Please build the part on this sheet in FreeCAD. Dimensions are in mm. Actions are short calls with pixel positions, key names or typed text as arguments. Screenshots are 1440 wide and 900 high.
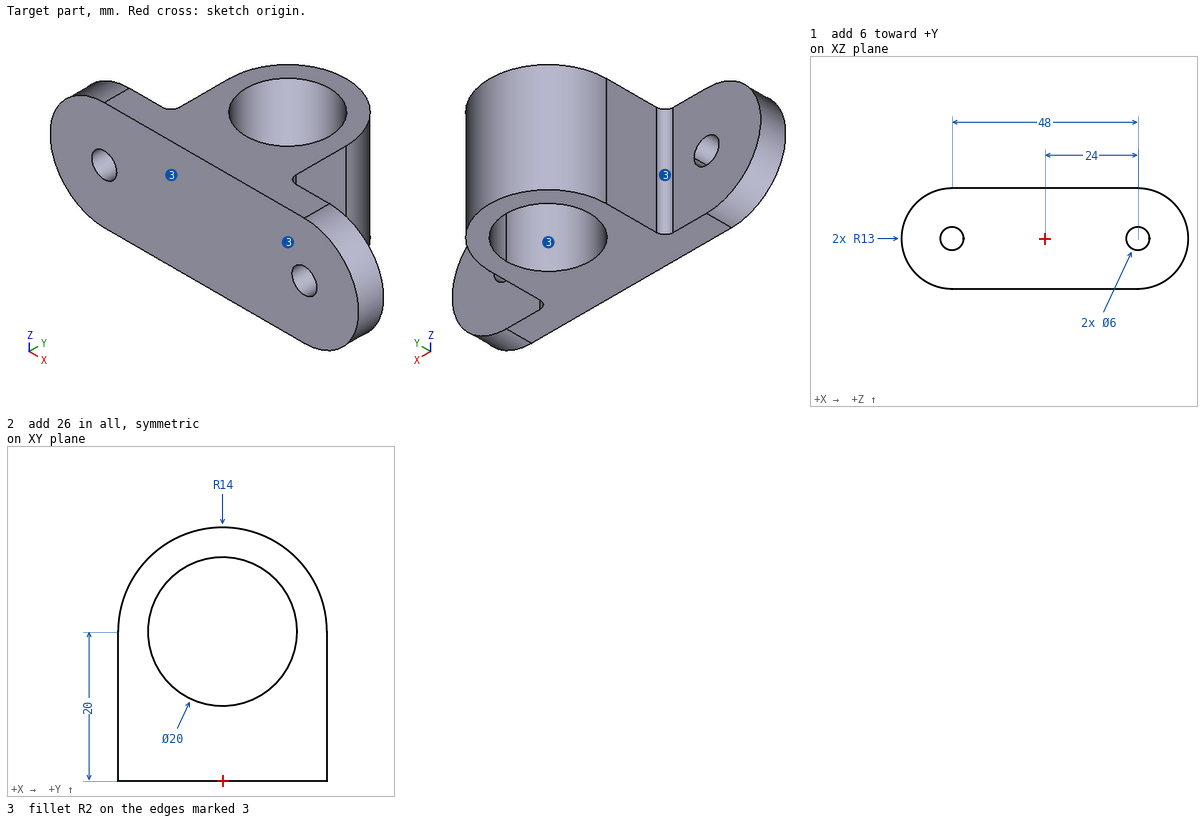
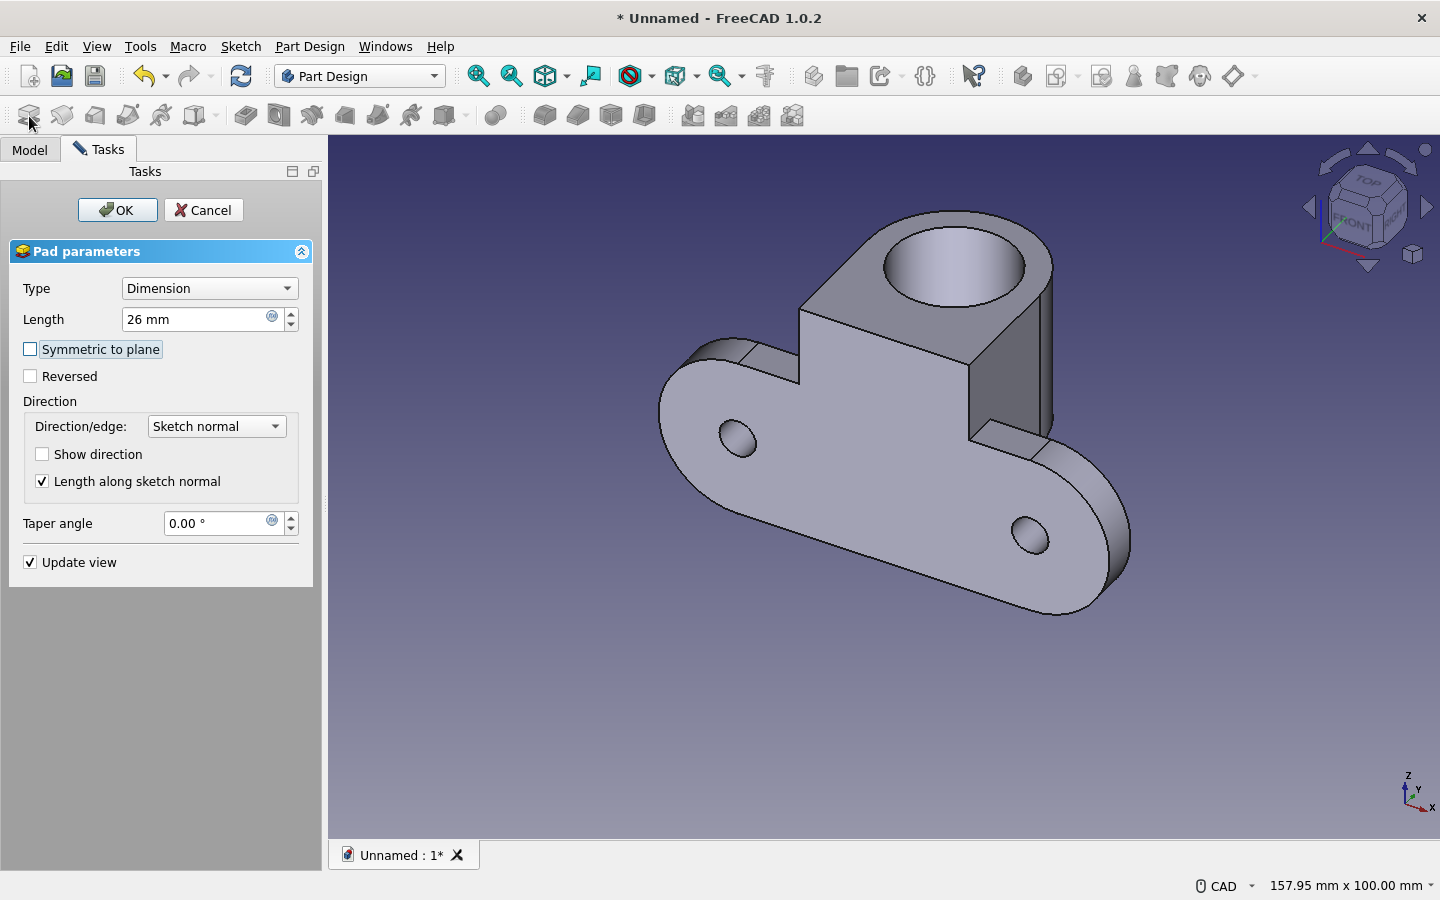
click(31, 349)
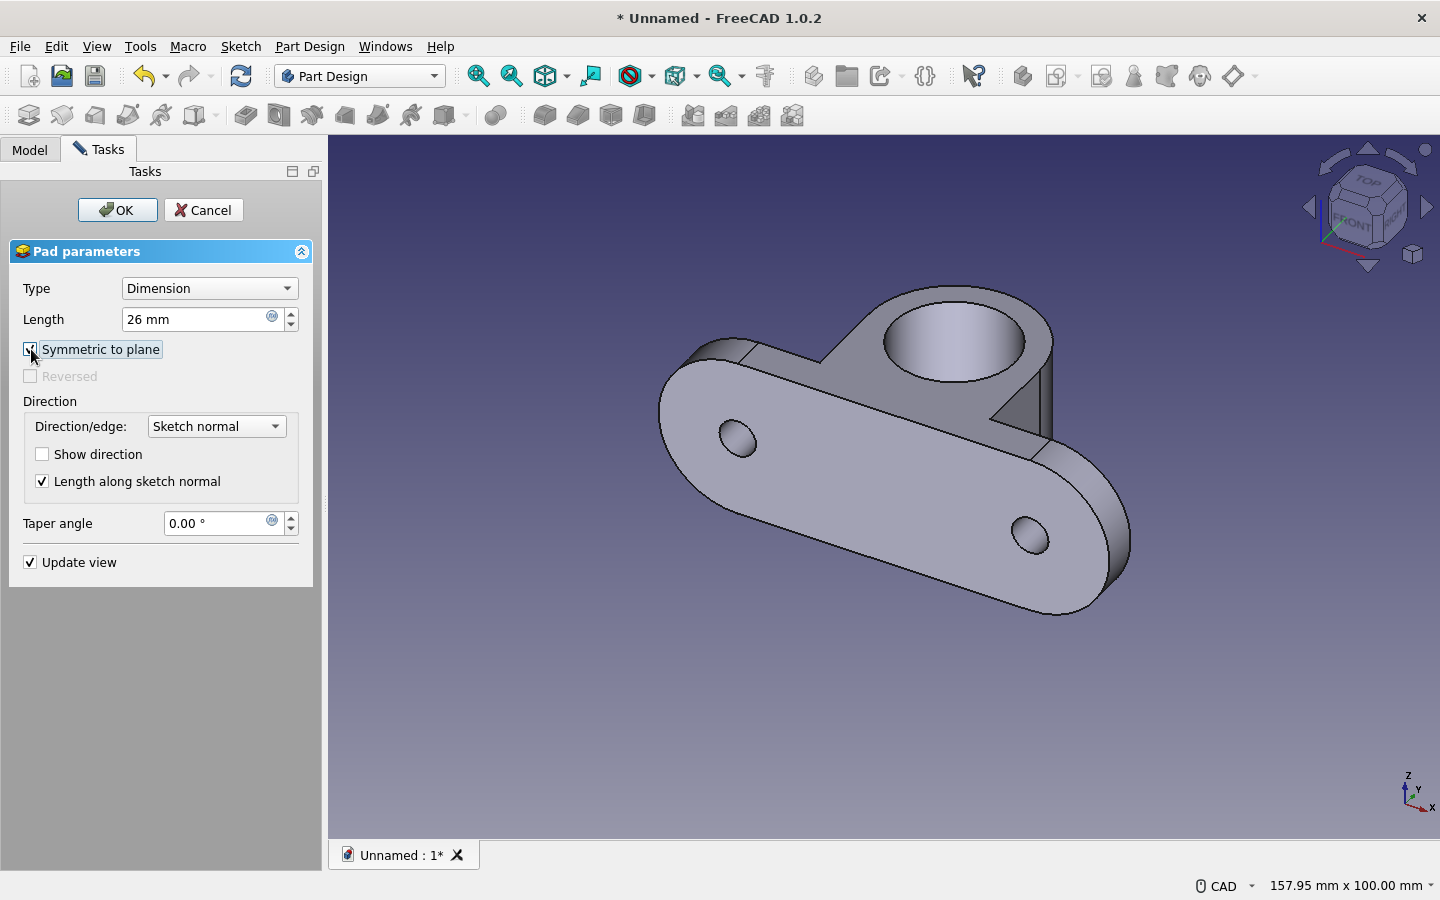
click(118, 210)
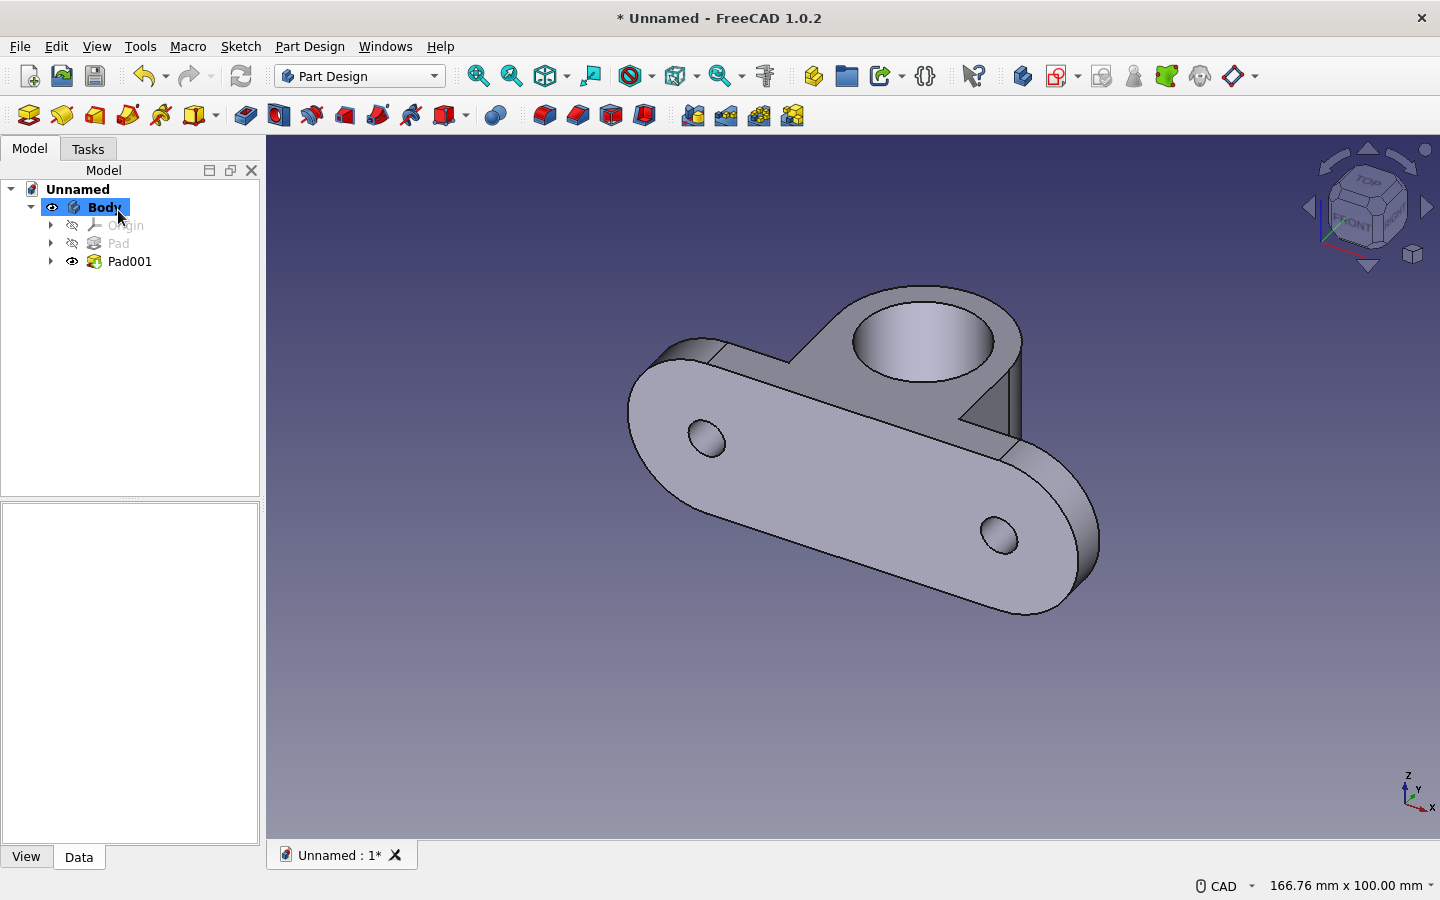
key(0)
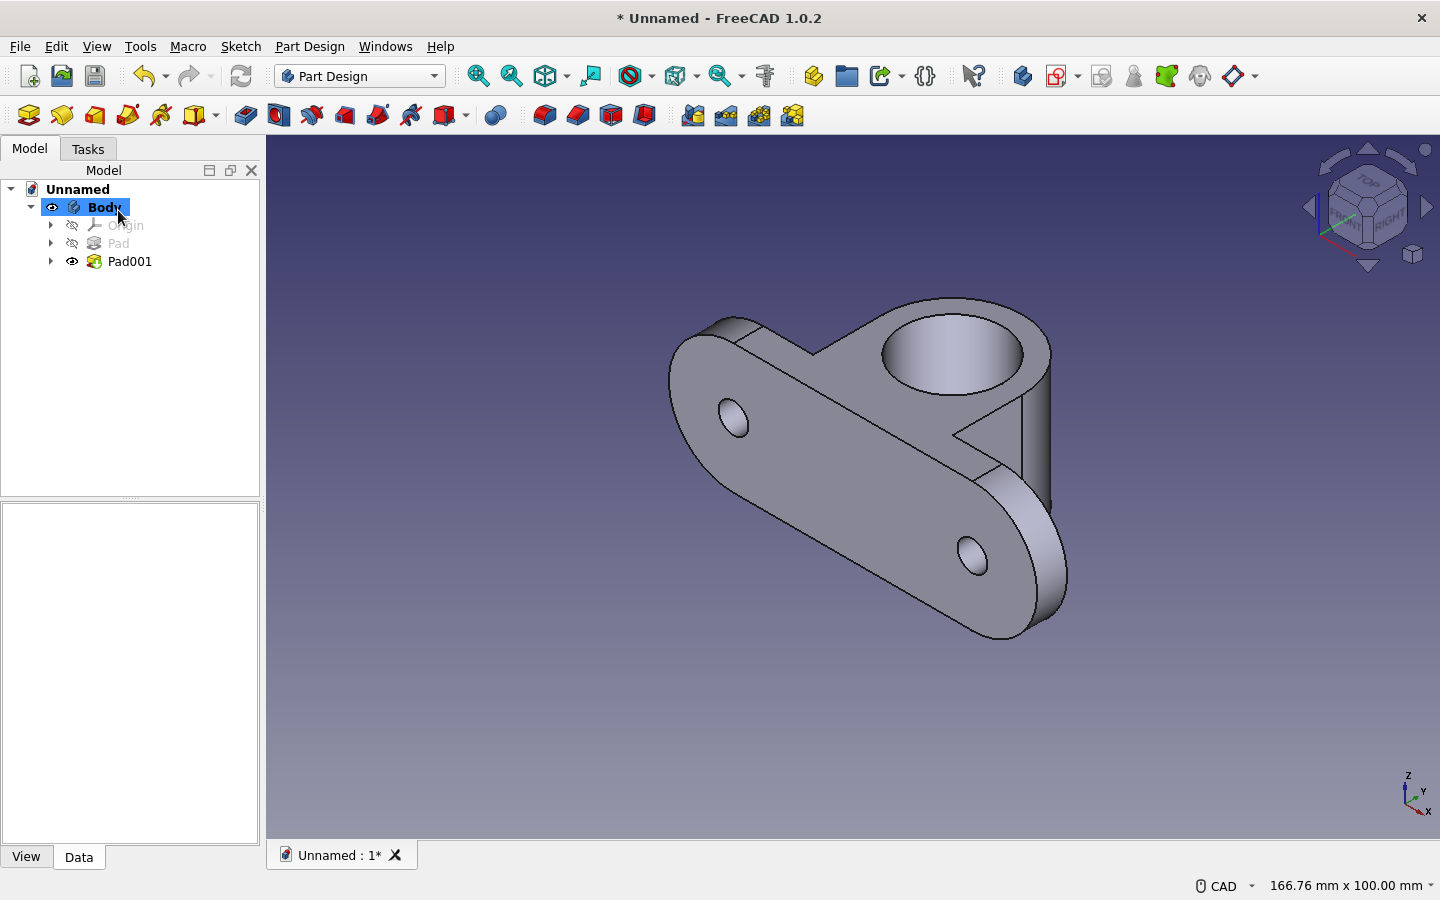
key(2)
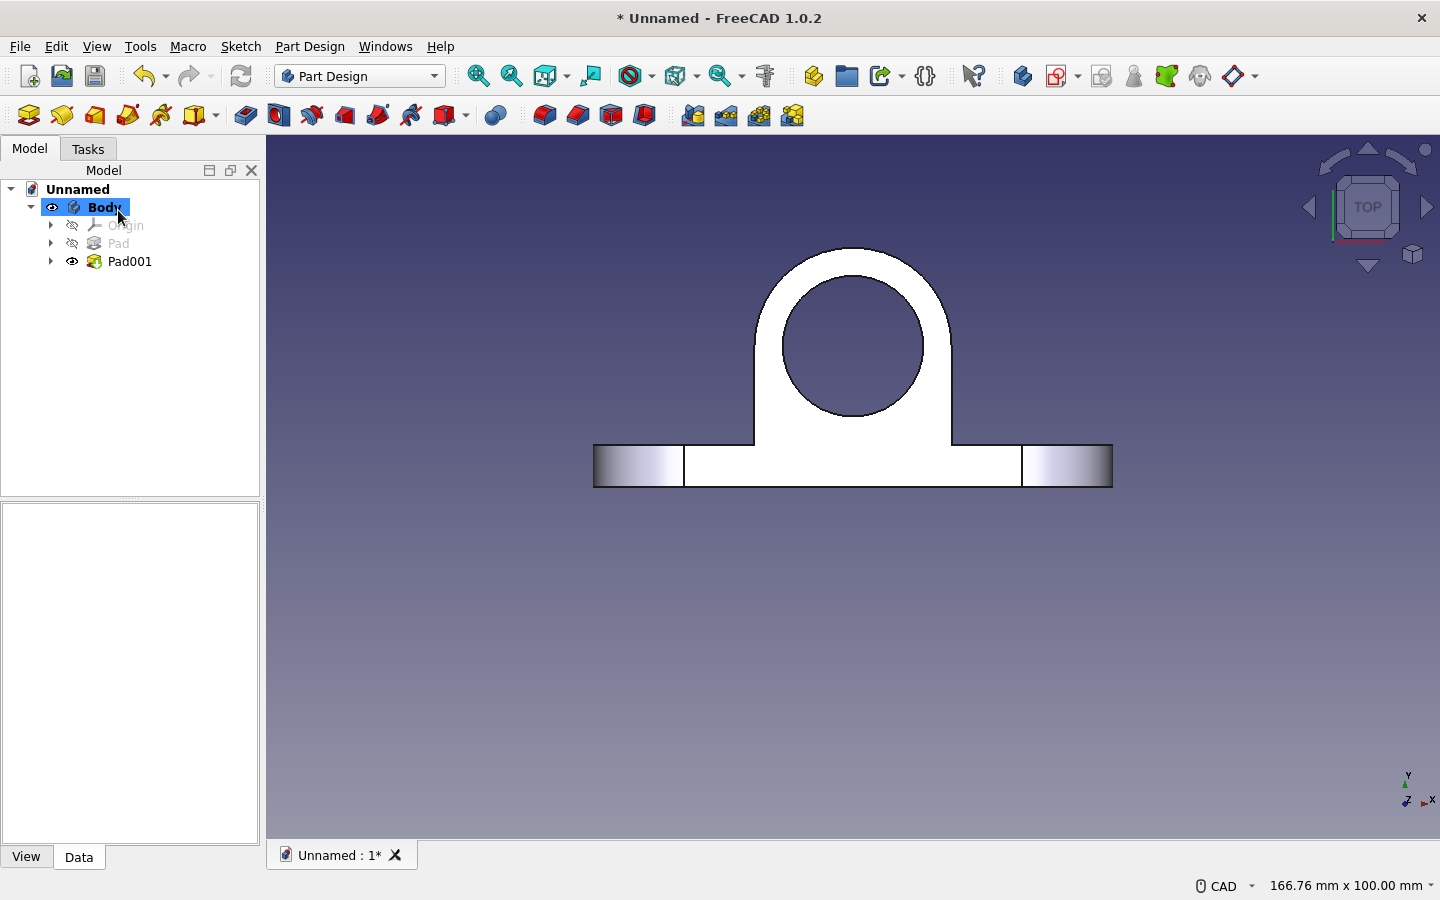
click(479, 76)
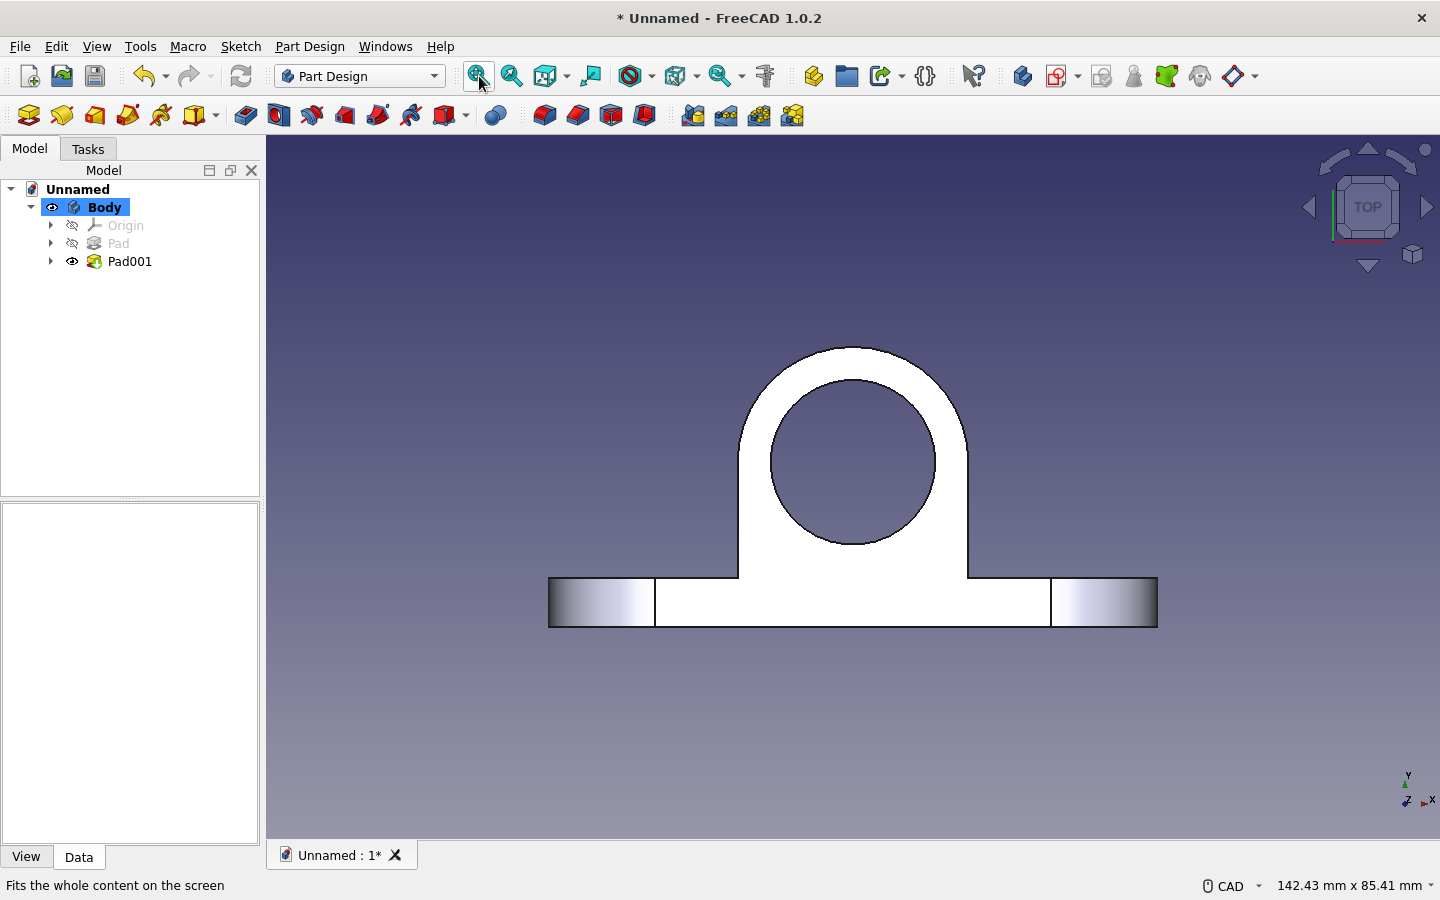
key(1)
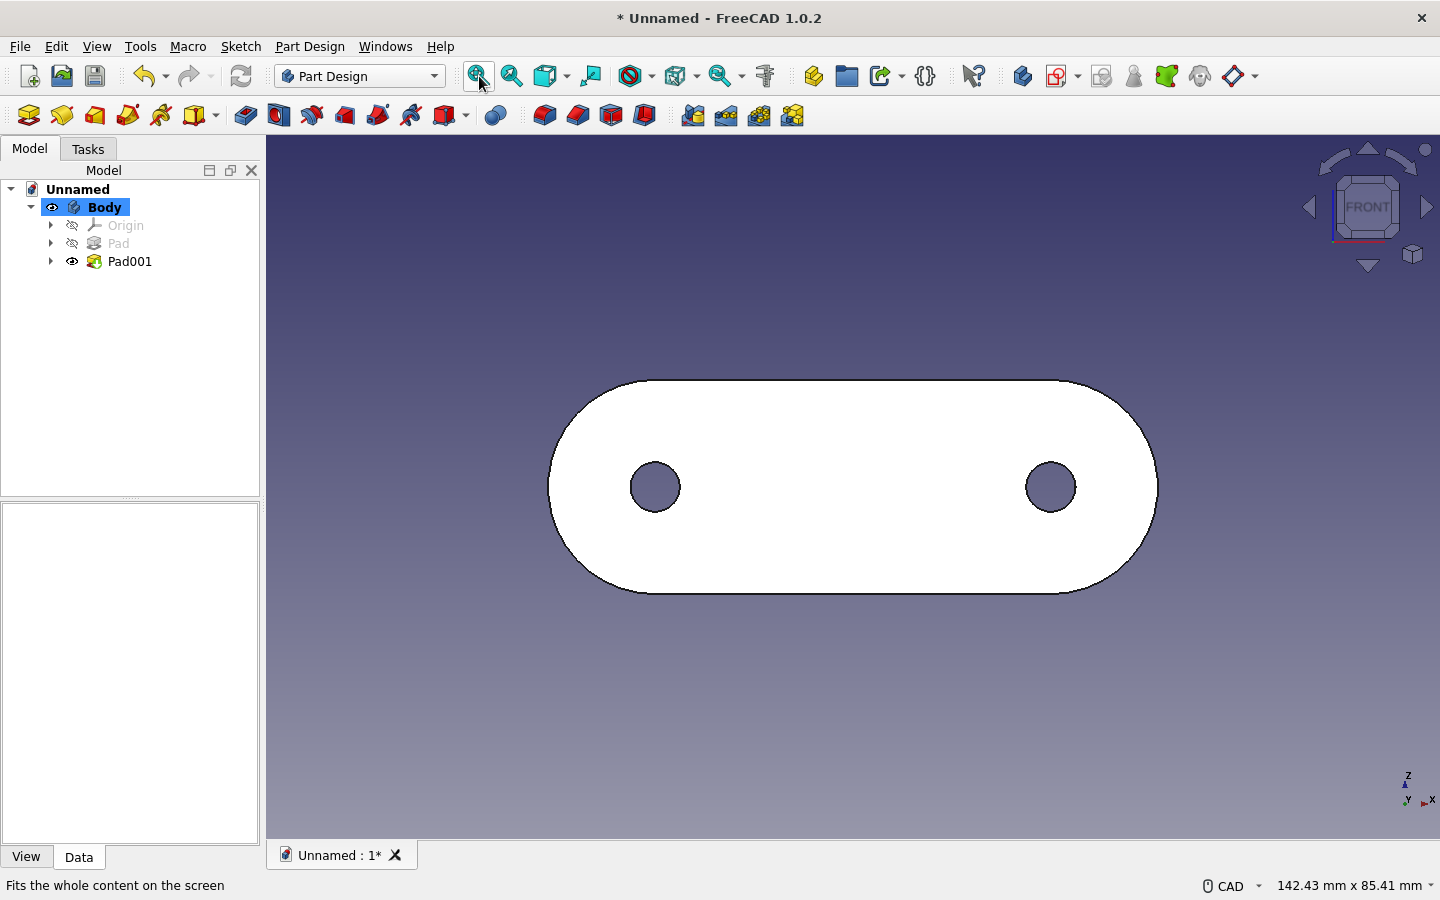
key(3)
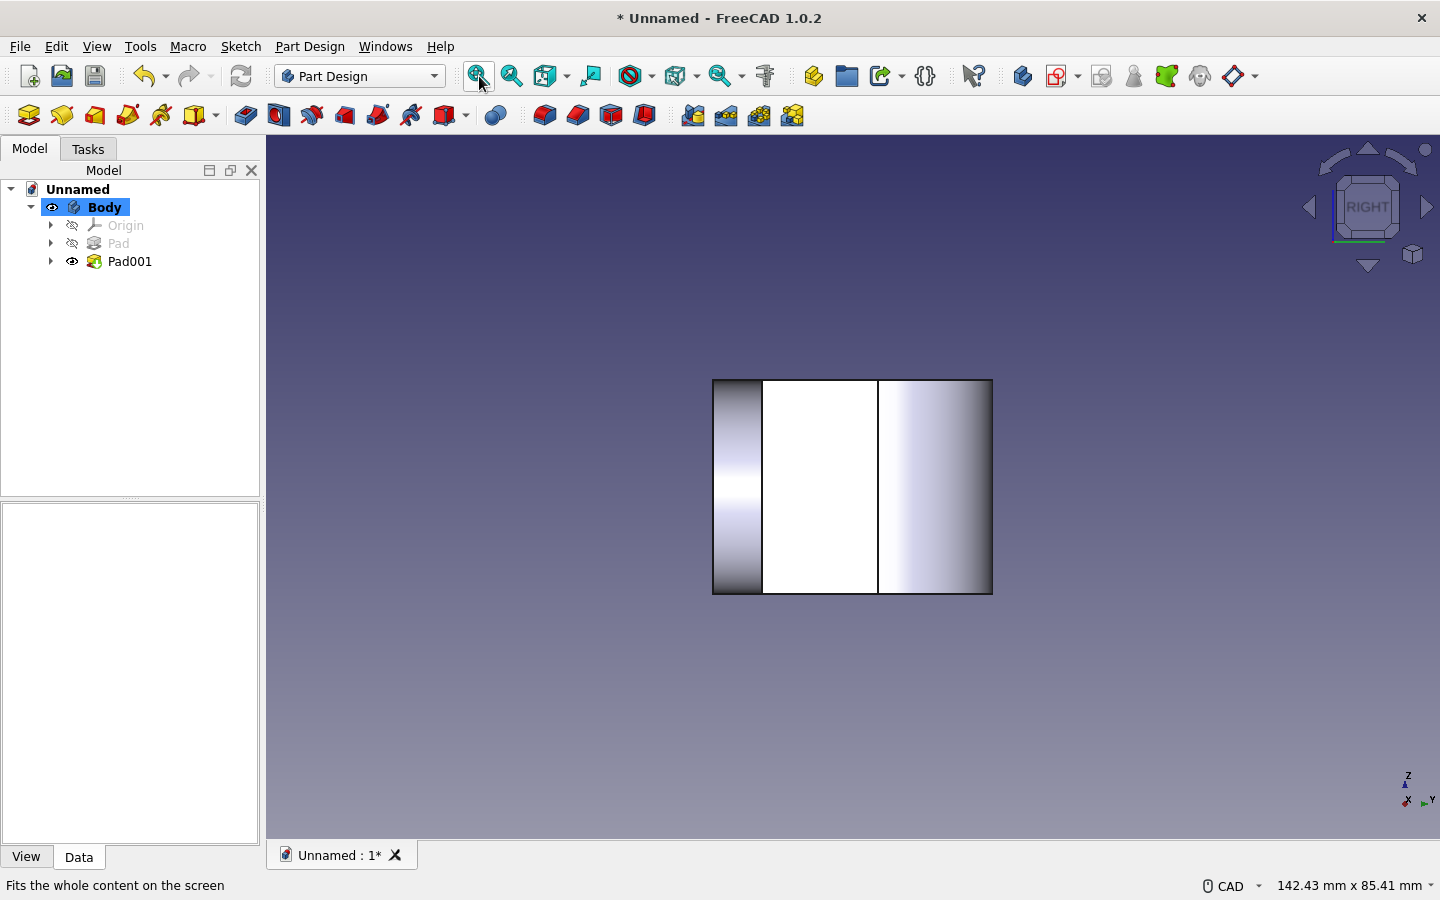
key(v)
key(f)